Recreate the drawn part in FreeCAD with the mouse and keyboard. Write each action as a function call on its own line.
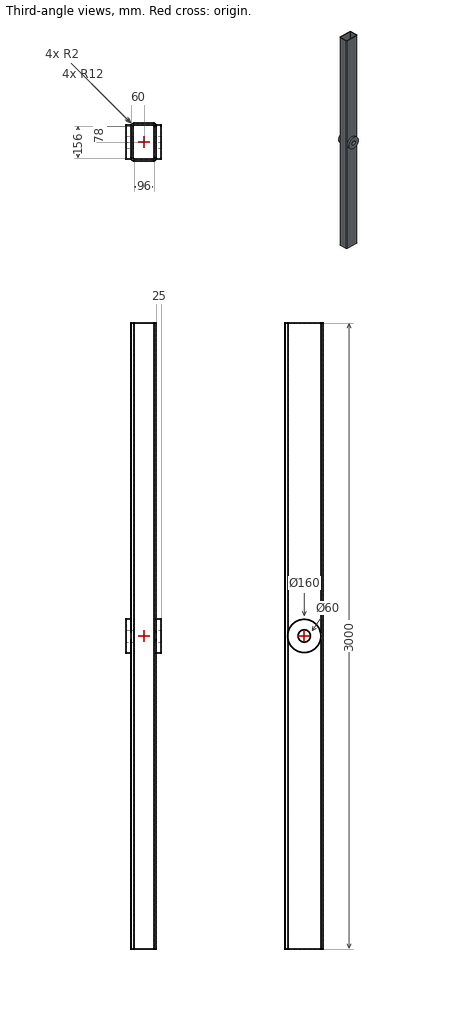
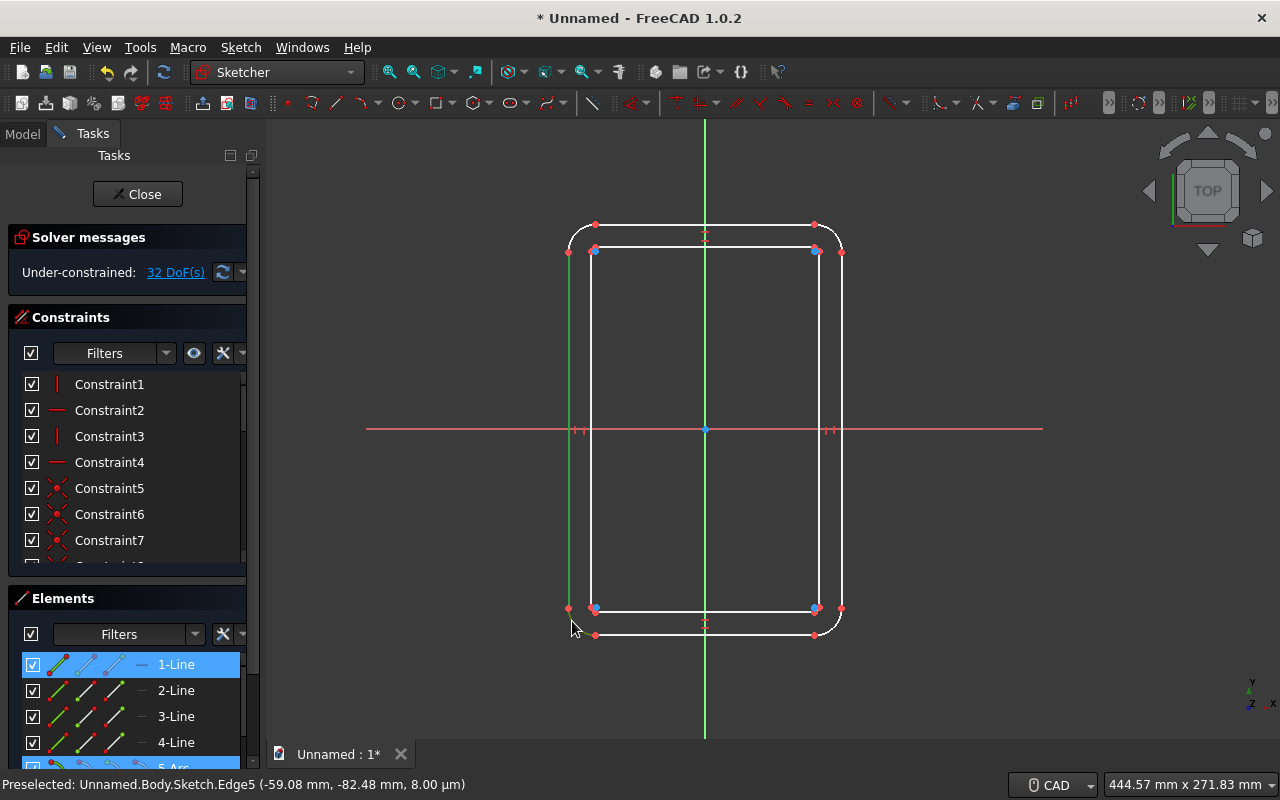
click(786, 104)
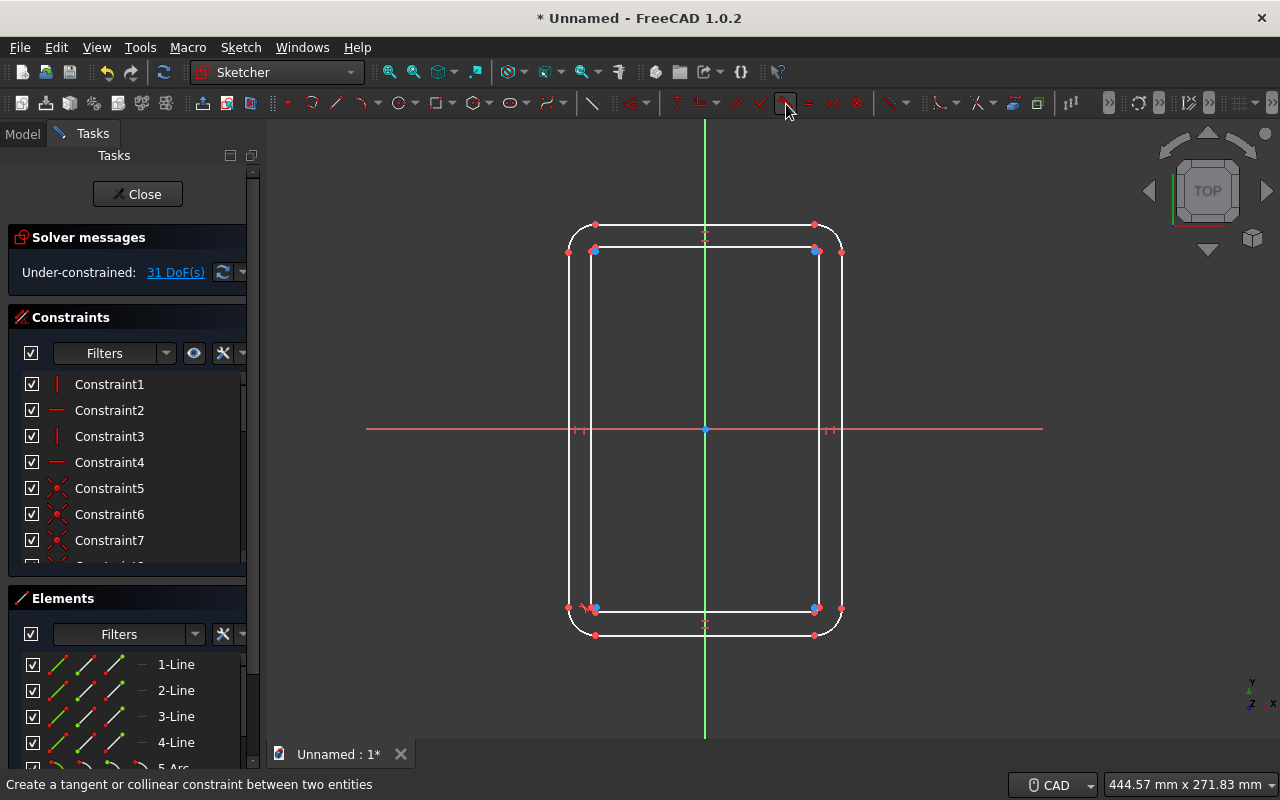
click(569, 359)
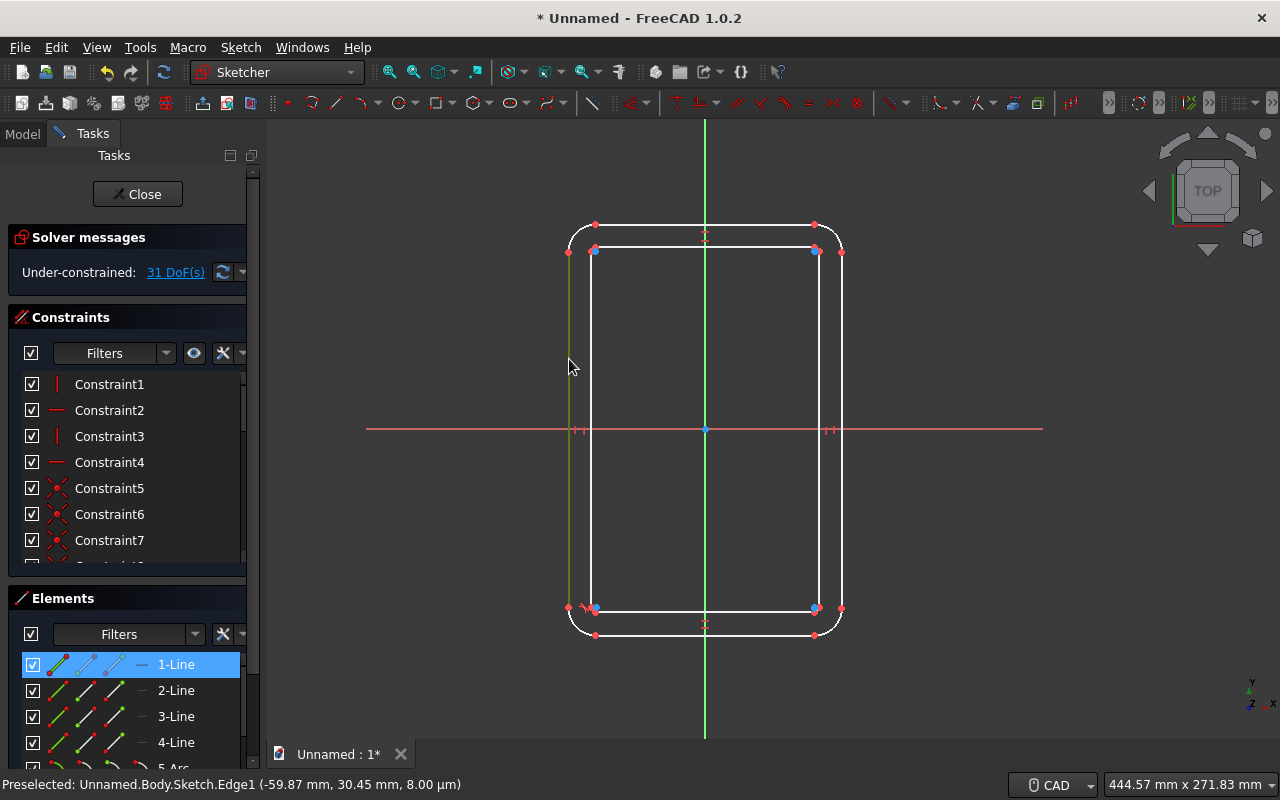
click(583, 228)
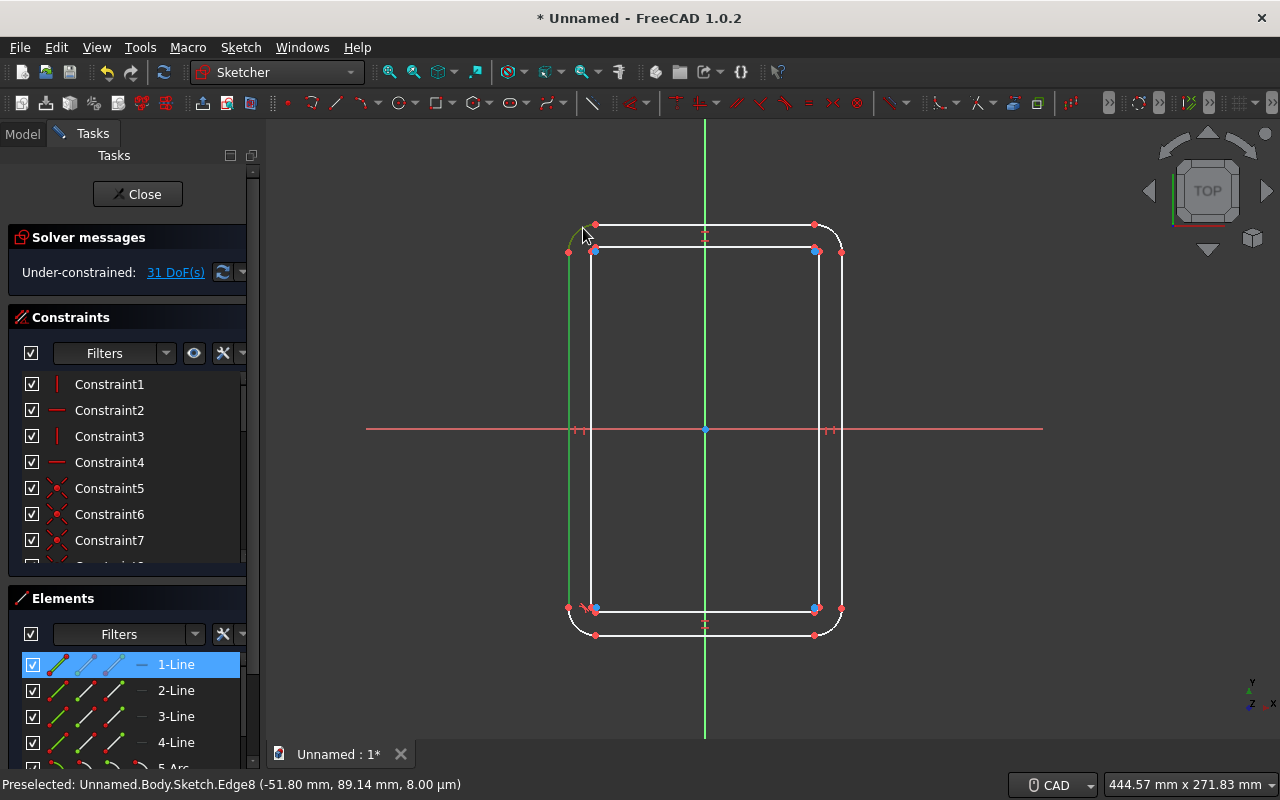
click(786, 104)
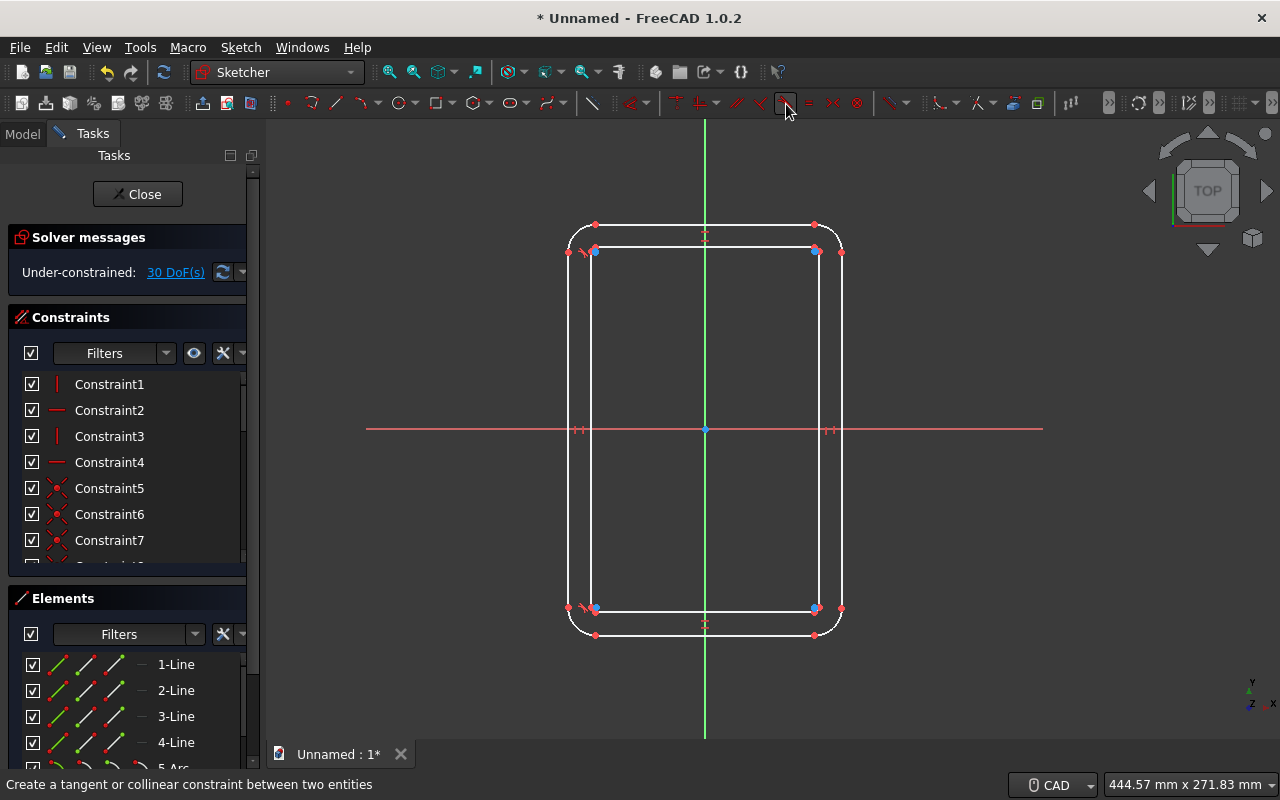
click(661, 636)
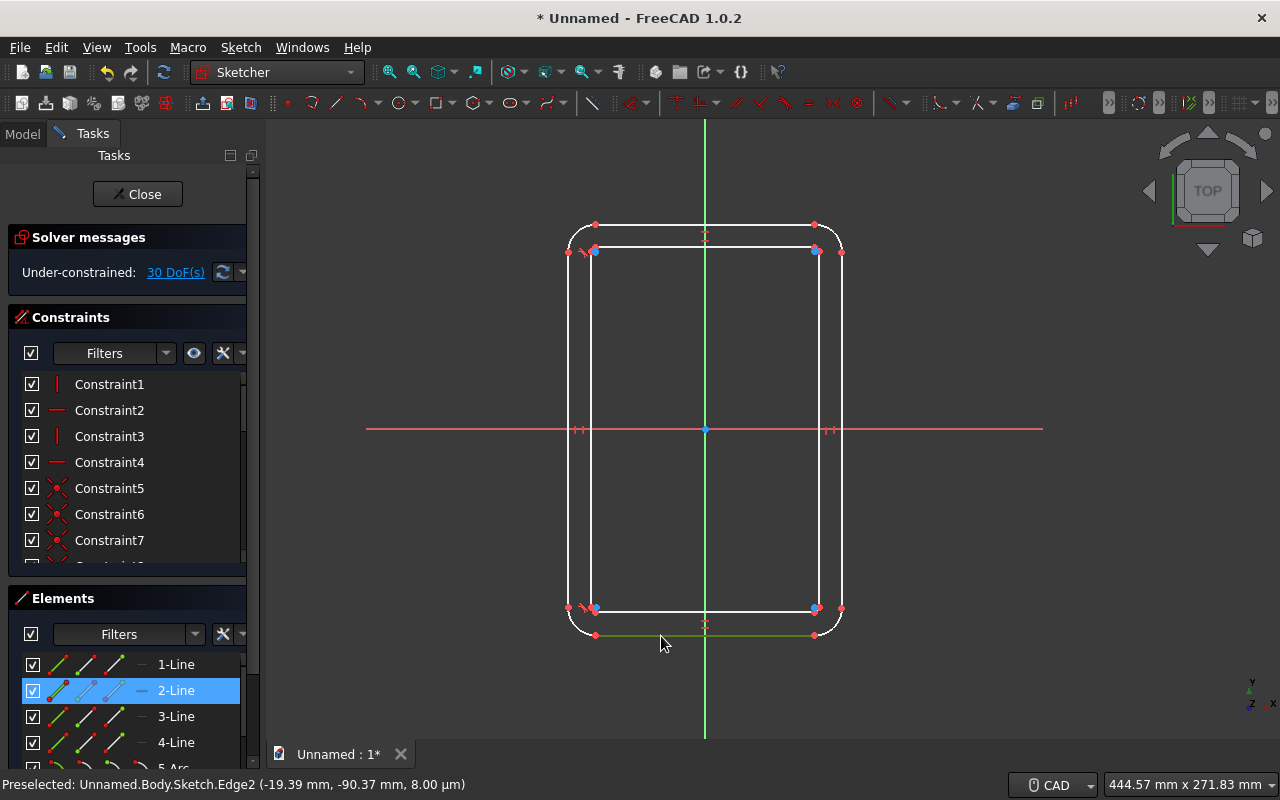
click(571, 620)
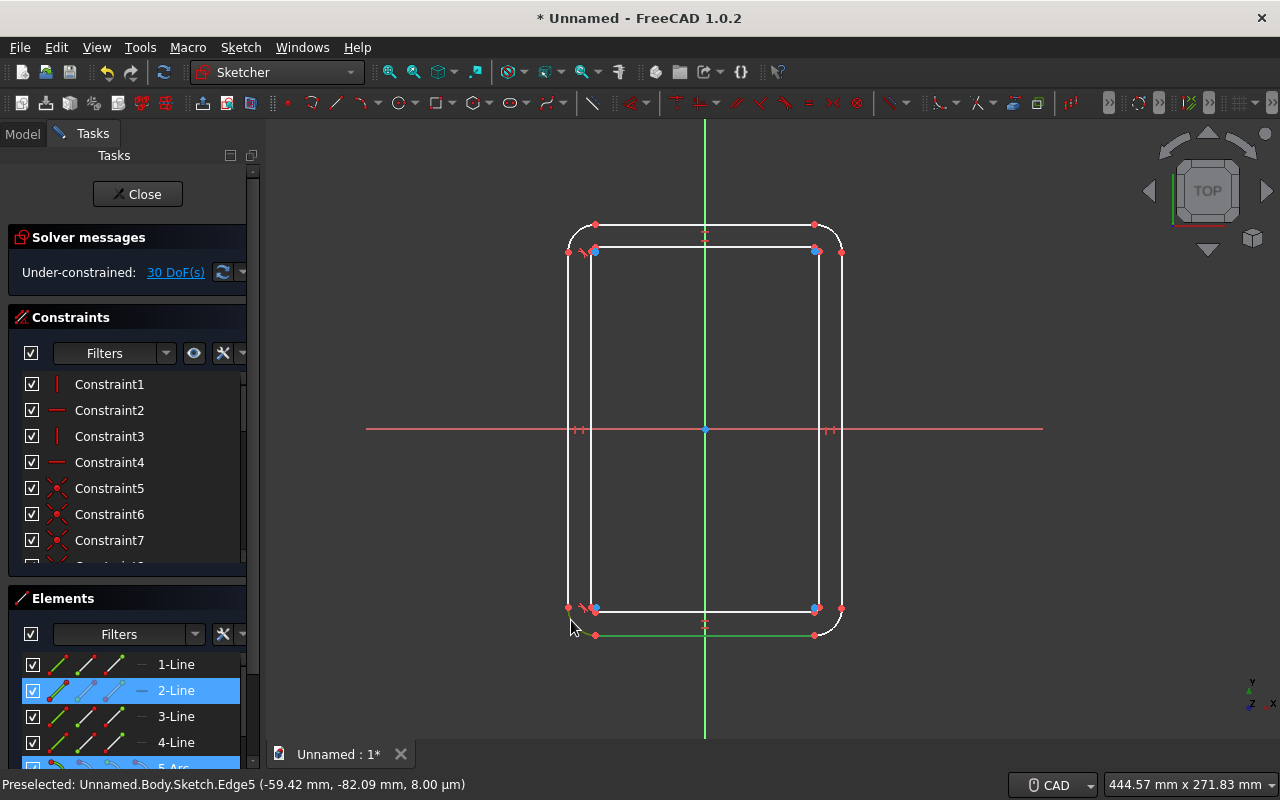
click(786, 104)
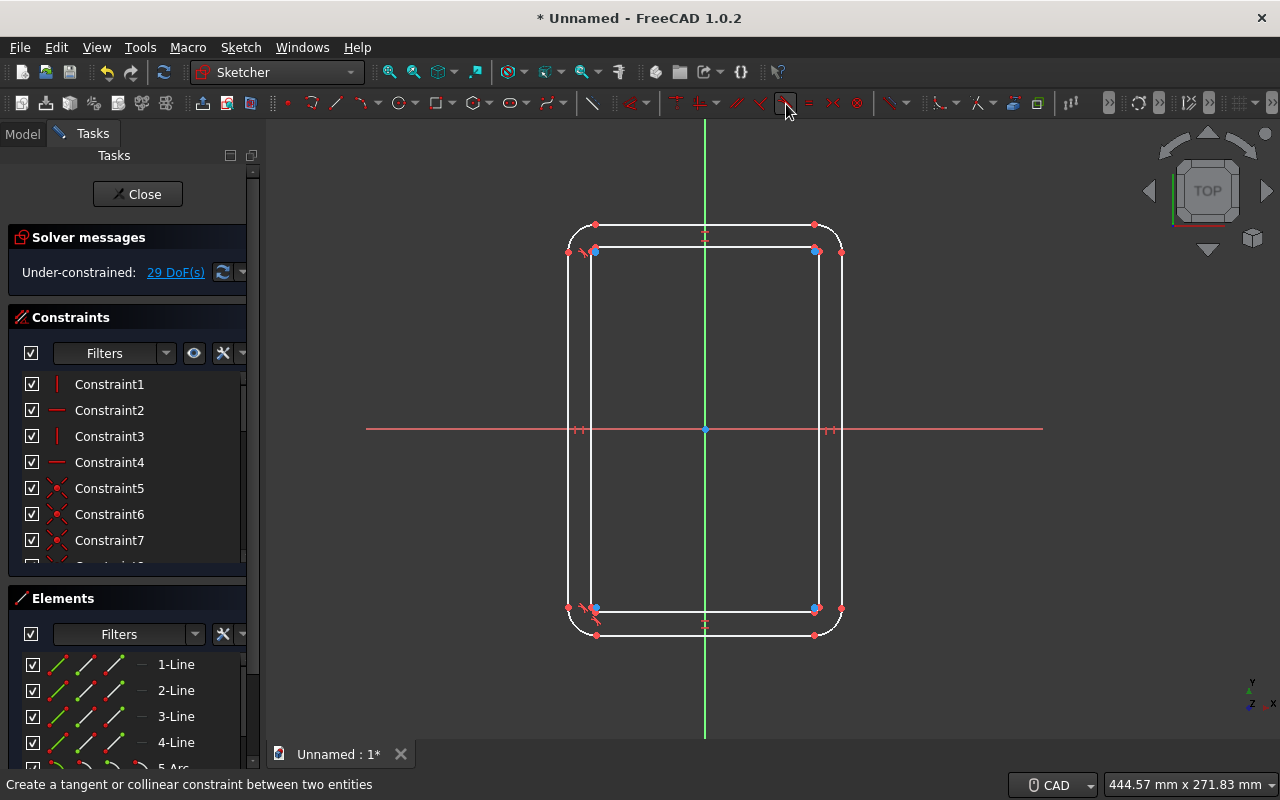
click(662, 636)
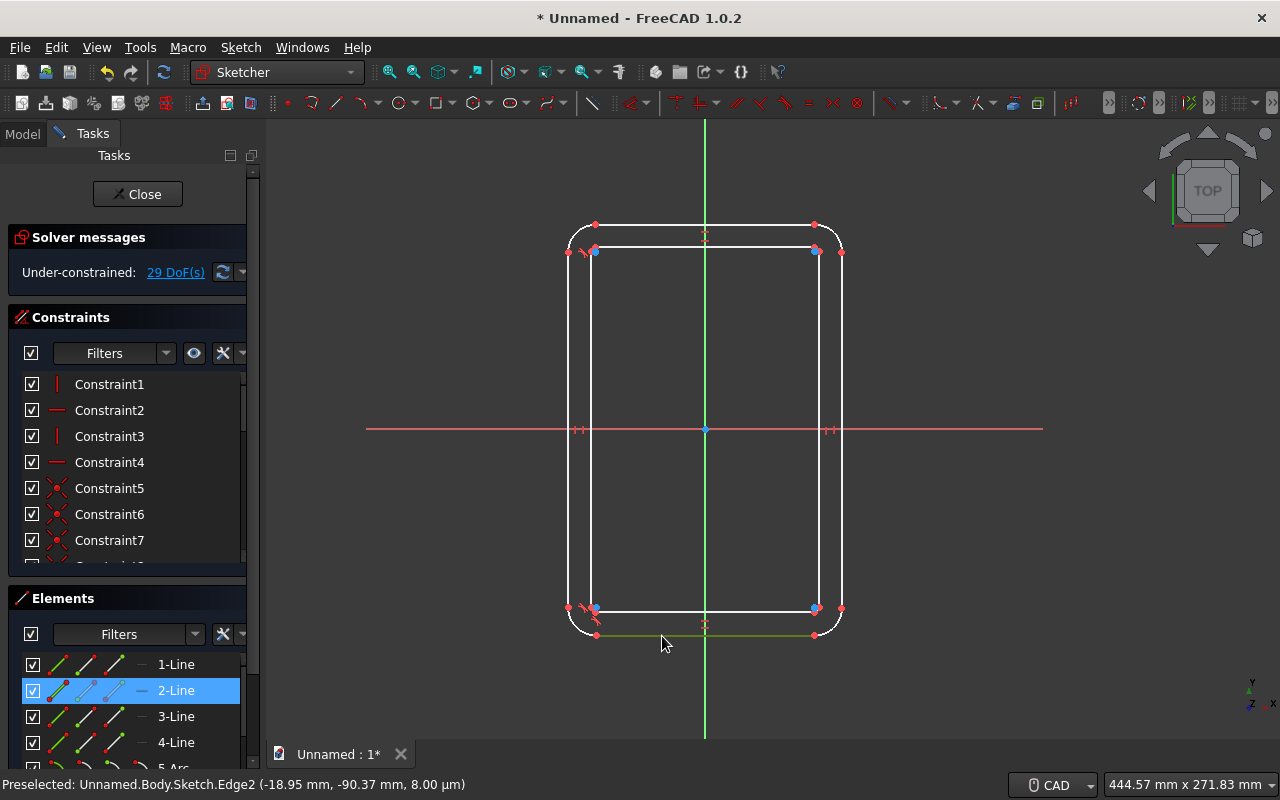
click(827, 632)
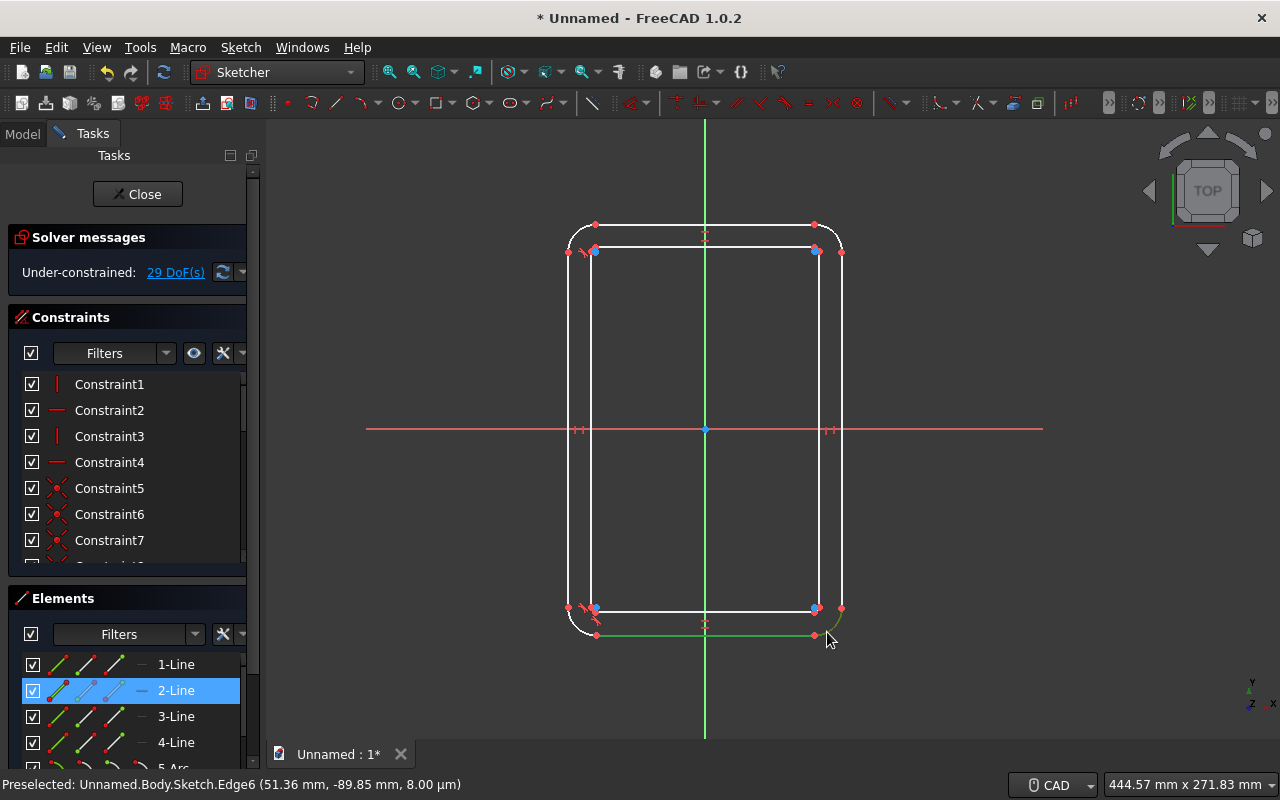
click(786, 104)